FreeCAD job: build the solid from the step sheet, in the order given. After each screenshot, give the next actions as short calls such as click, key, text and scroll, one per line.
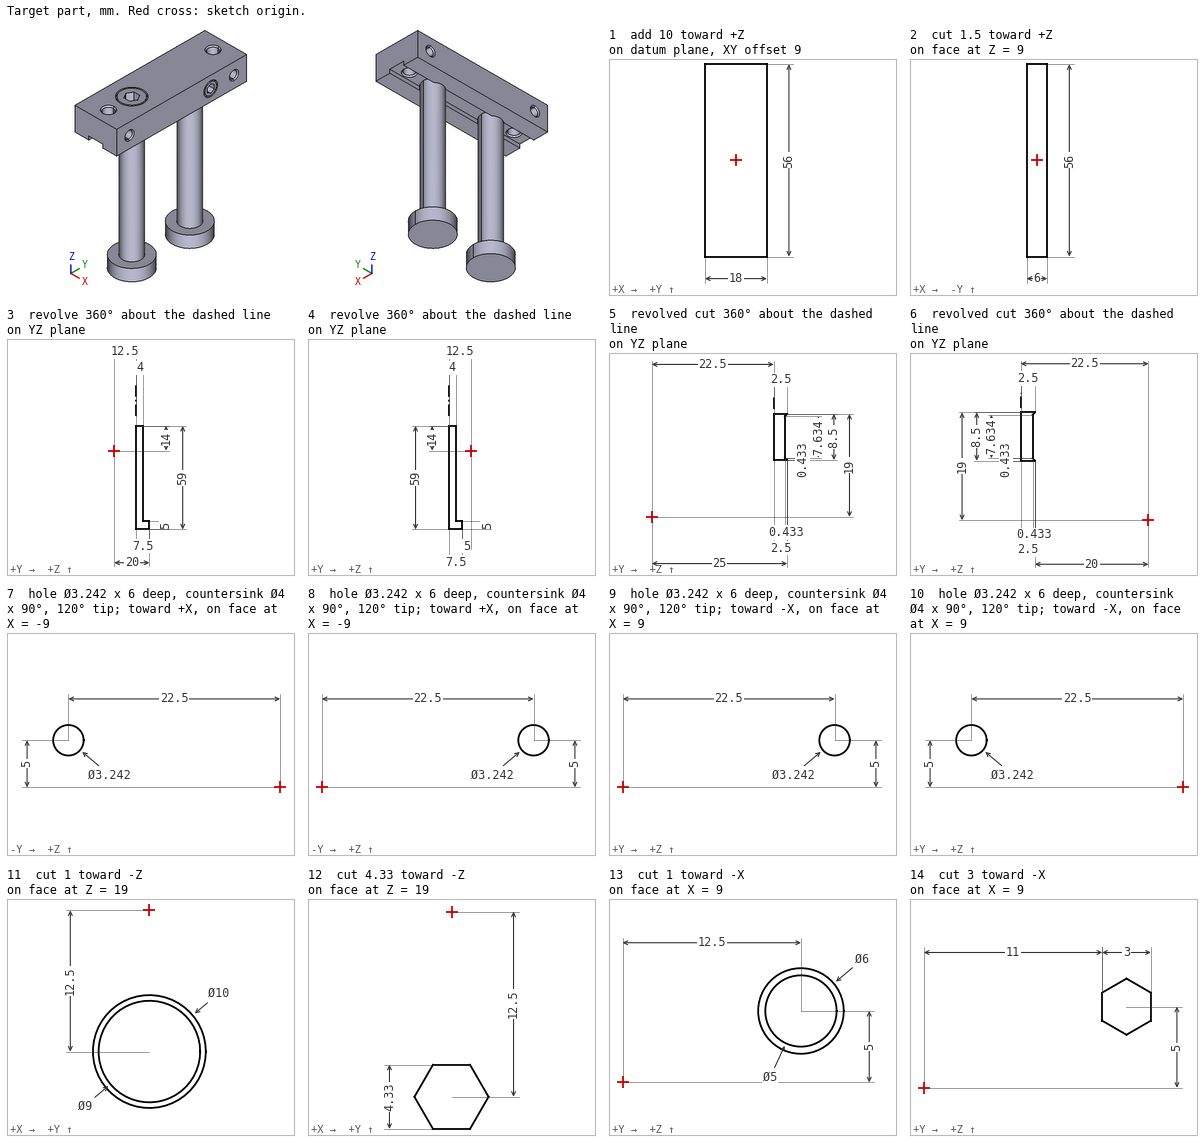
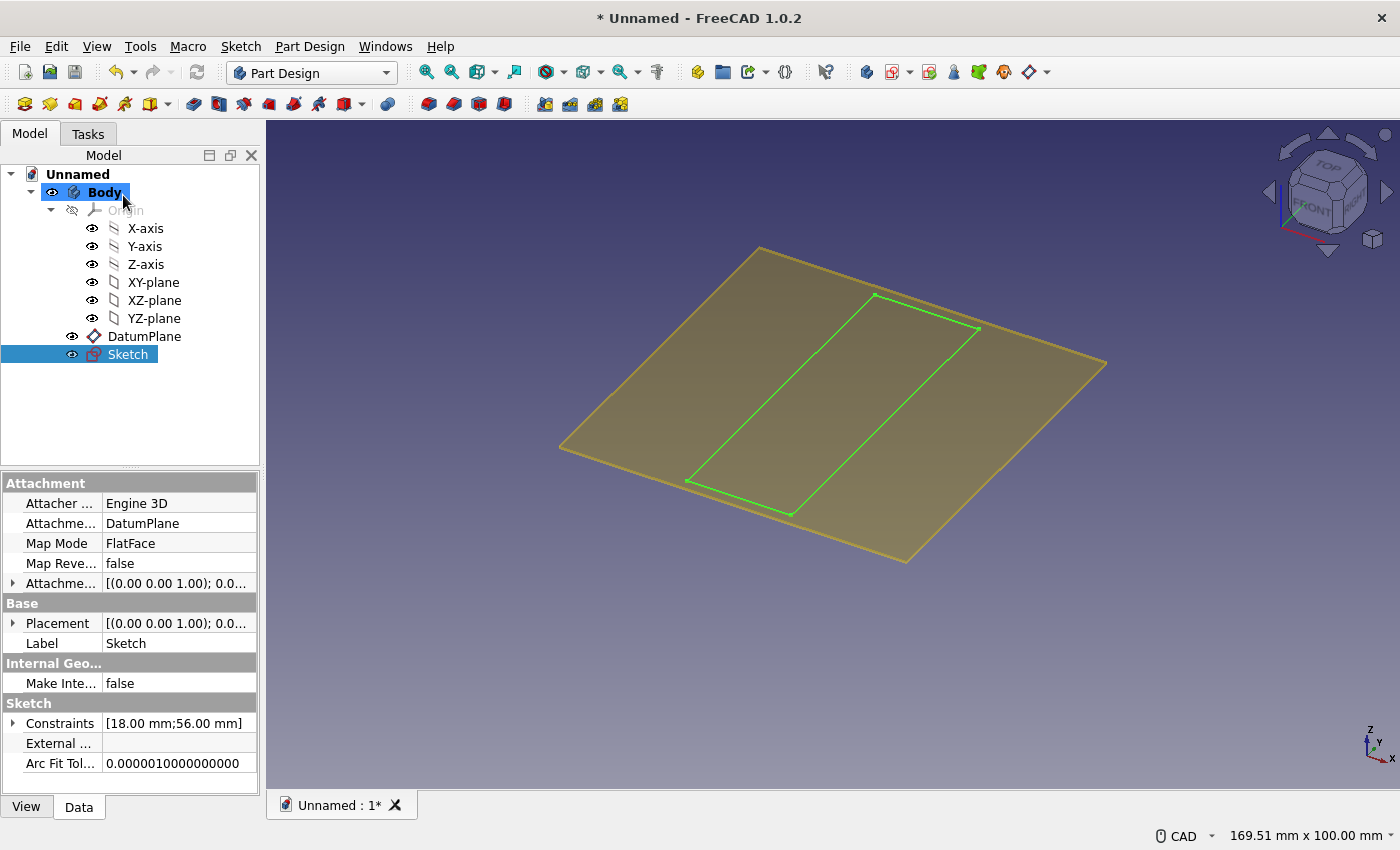
click(25, 104)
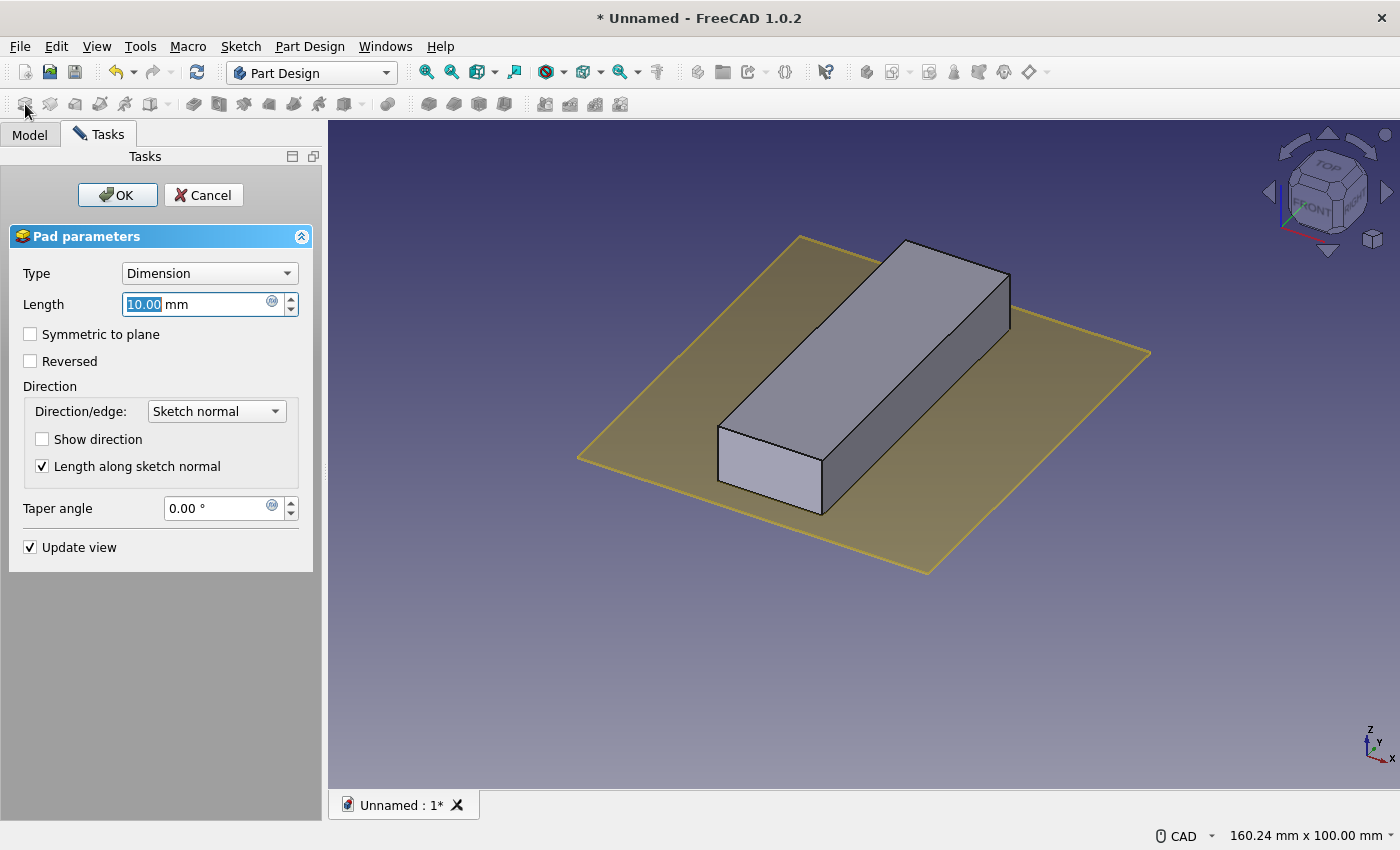
text(10)
key(Tab)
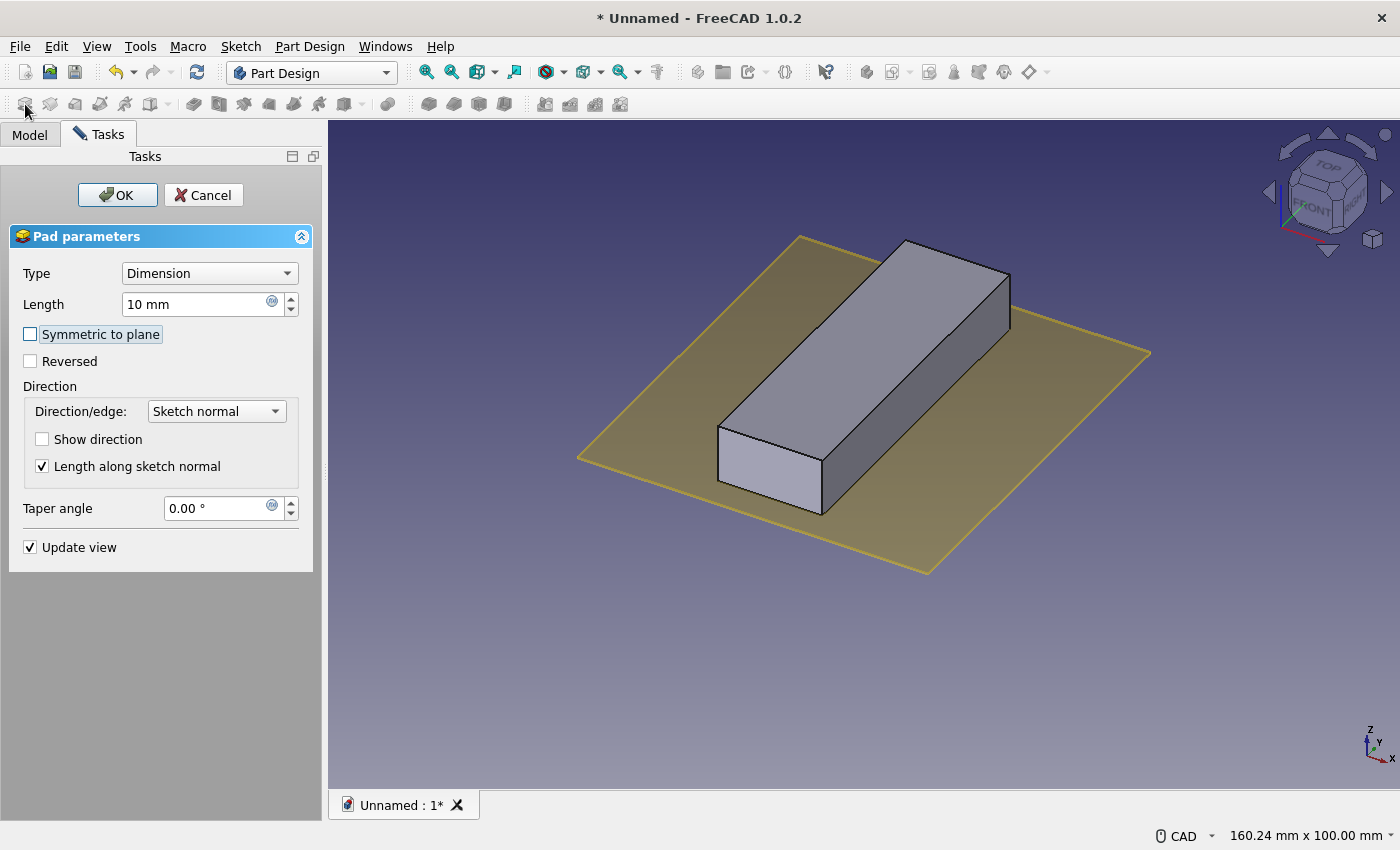
click(118, 195)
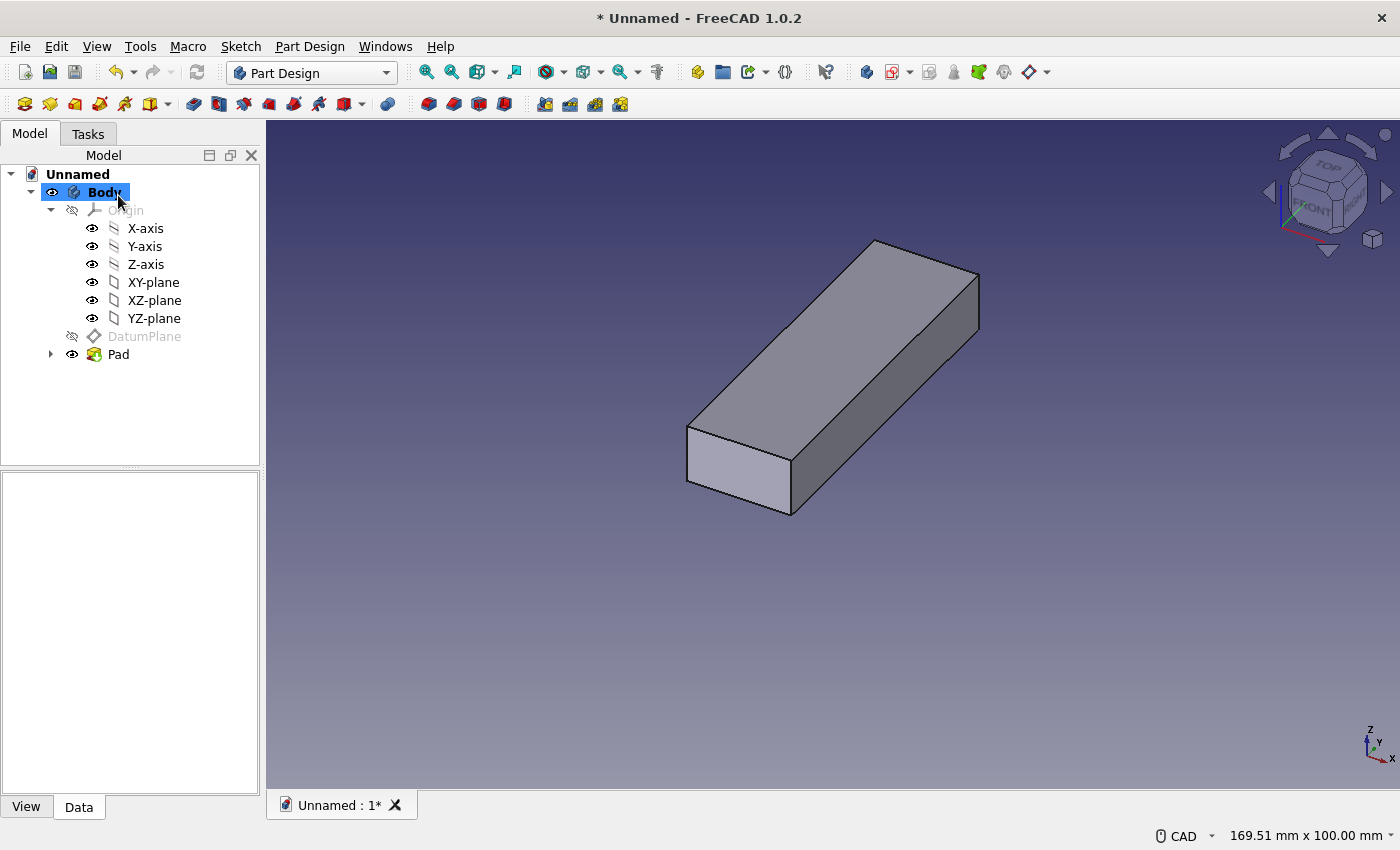
click(427, 72)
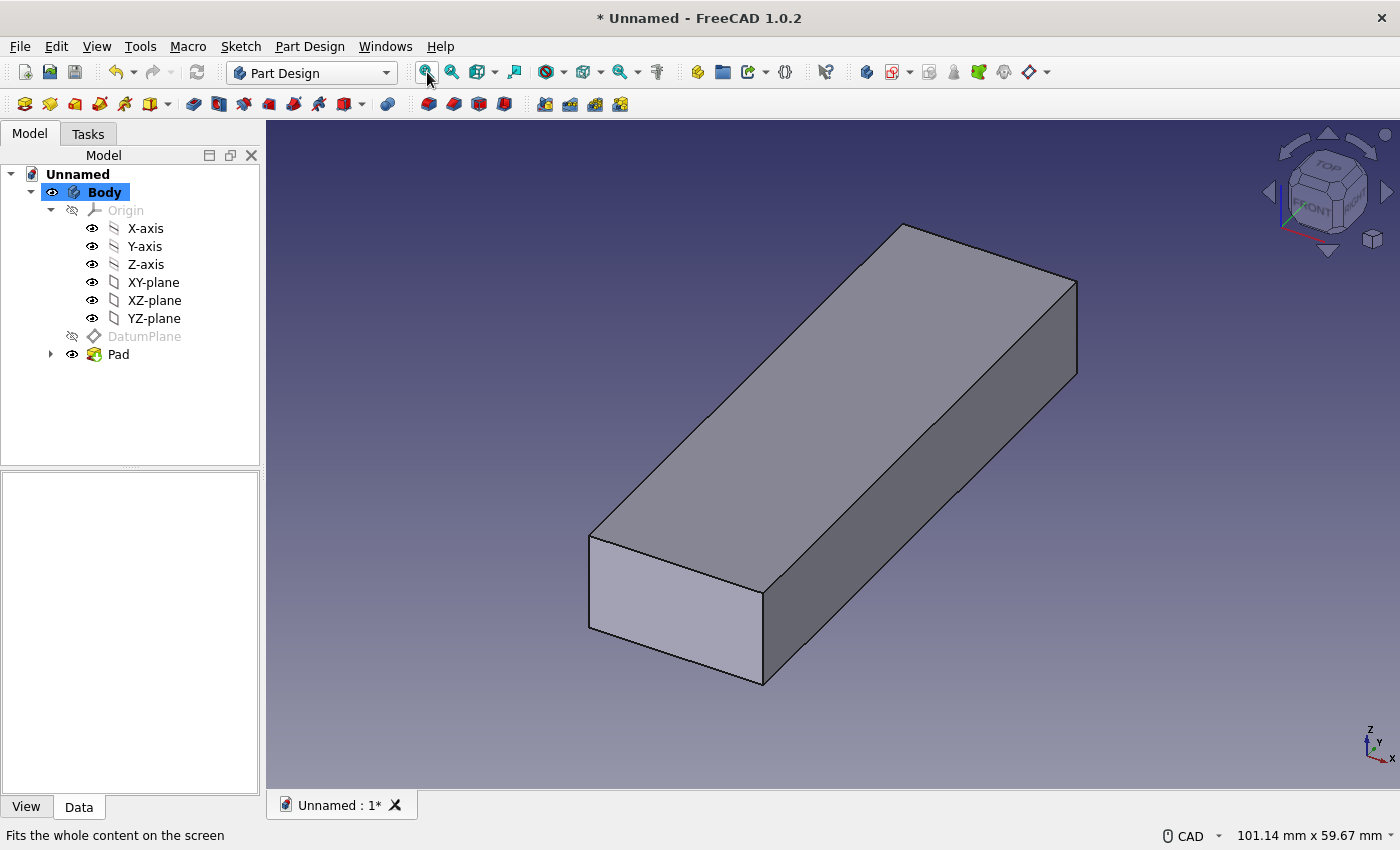
key(5)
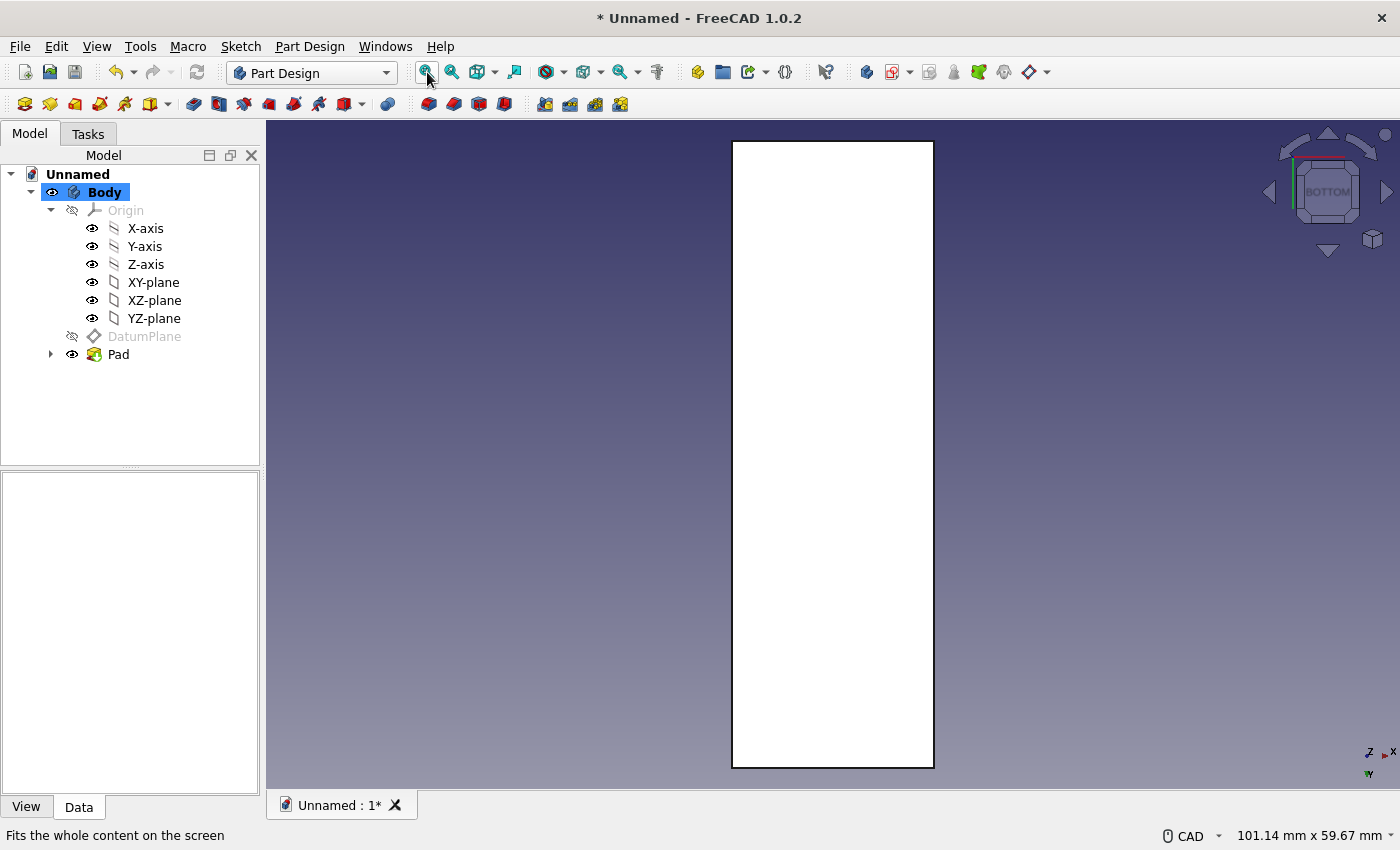
click(833, 633)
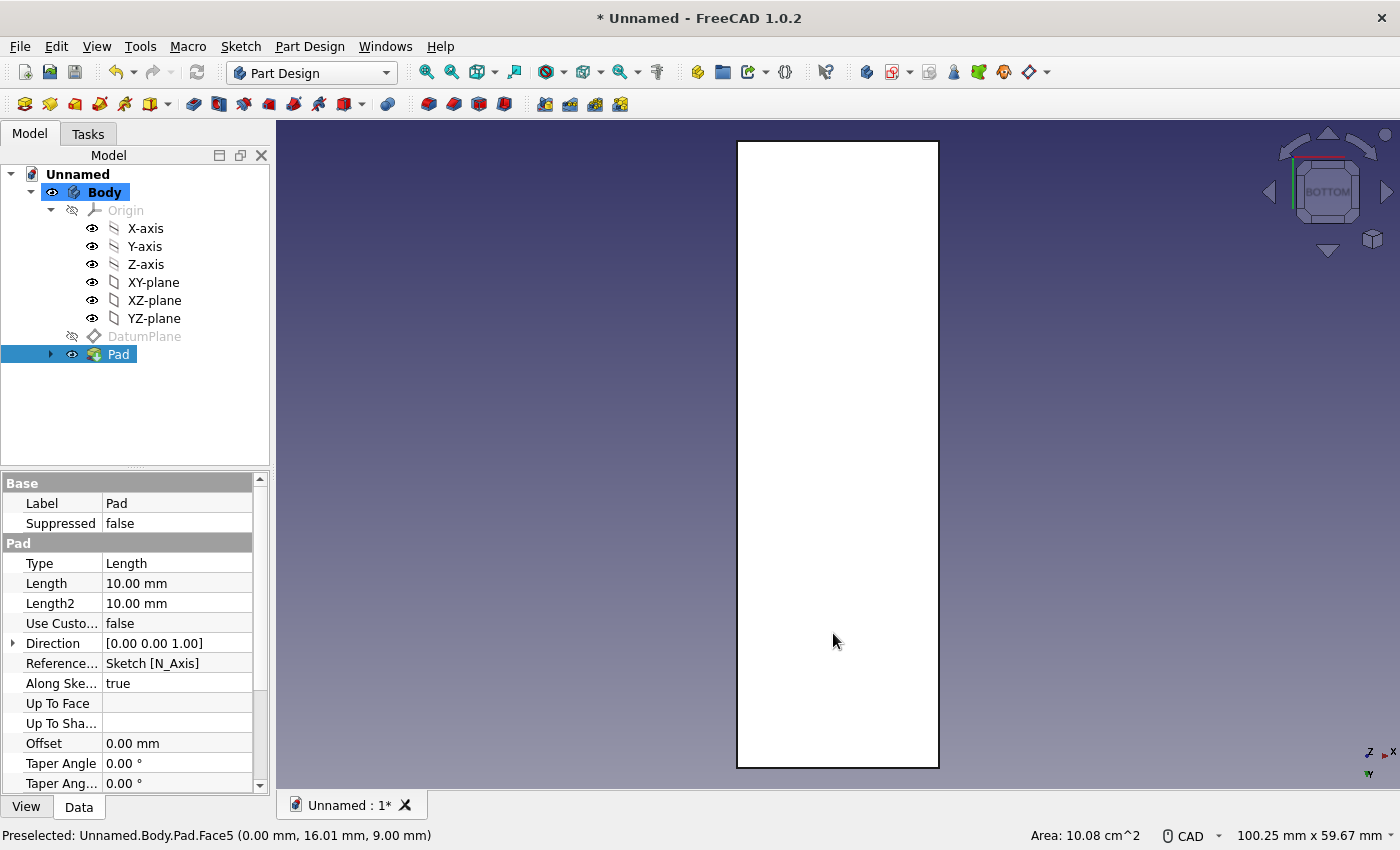
click(892, 72)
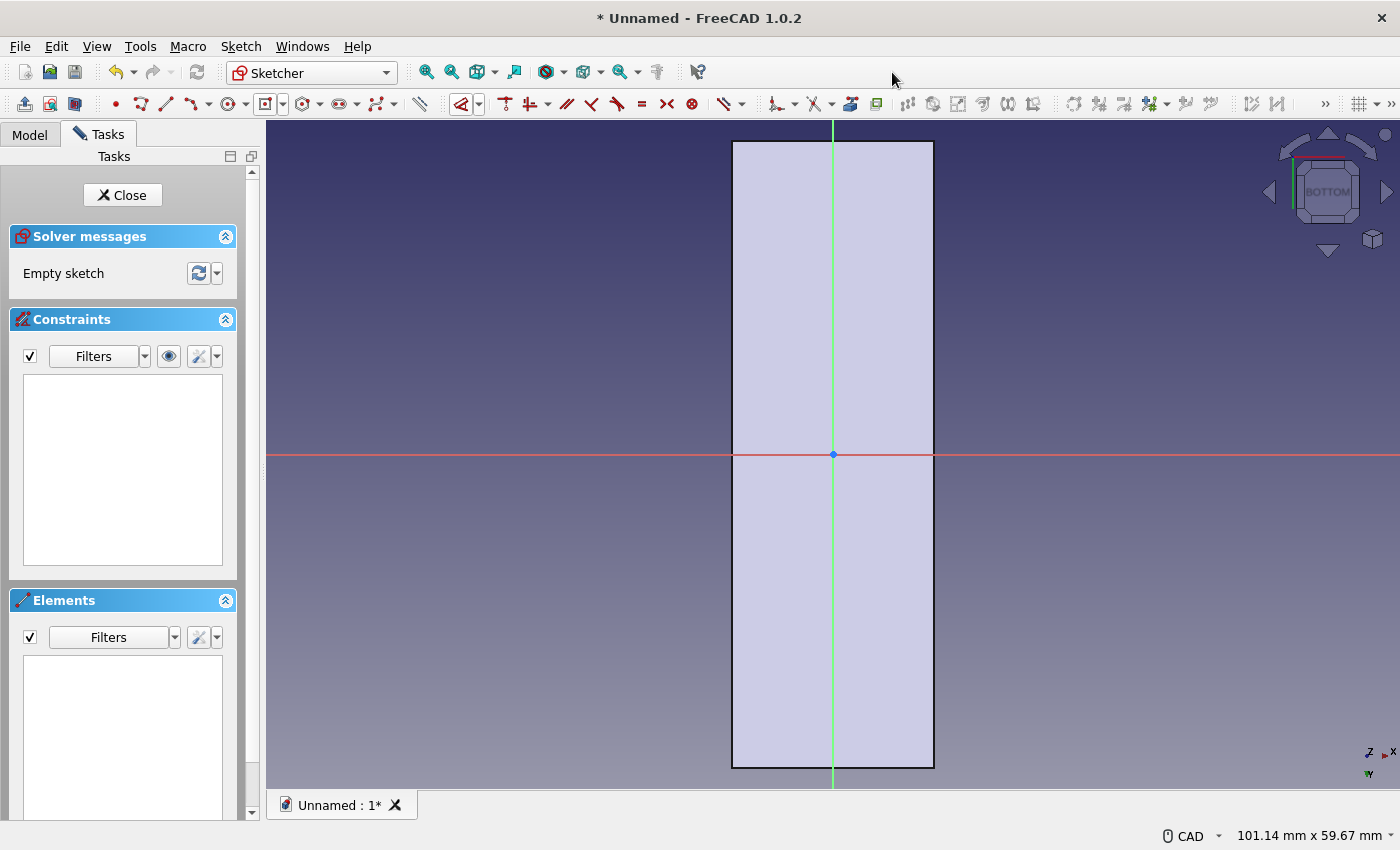
scroll(625, 455, down, 2)